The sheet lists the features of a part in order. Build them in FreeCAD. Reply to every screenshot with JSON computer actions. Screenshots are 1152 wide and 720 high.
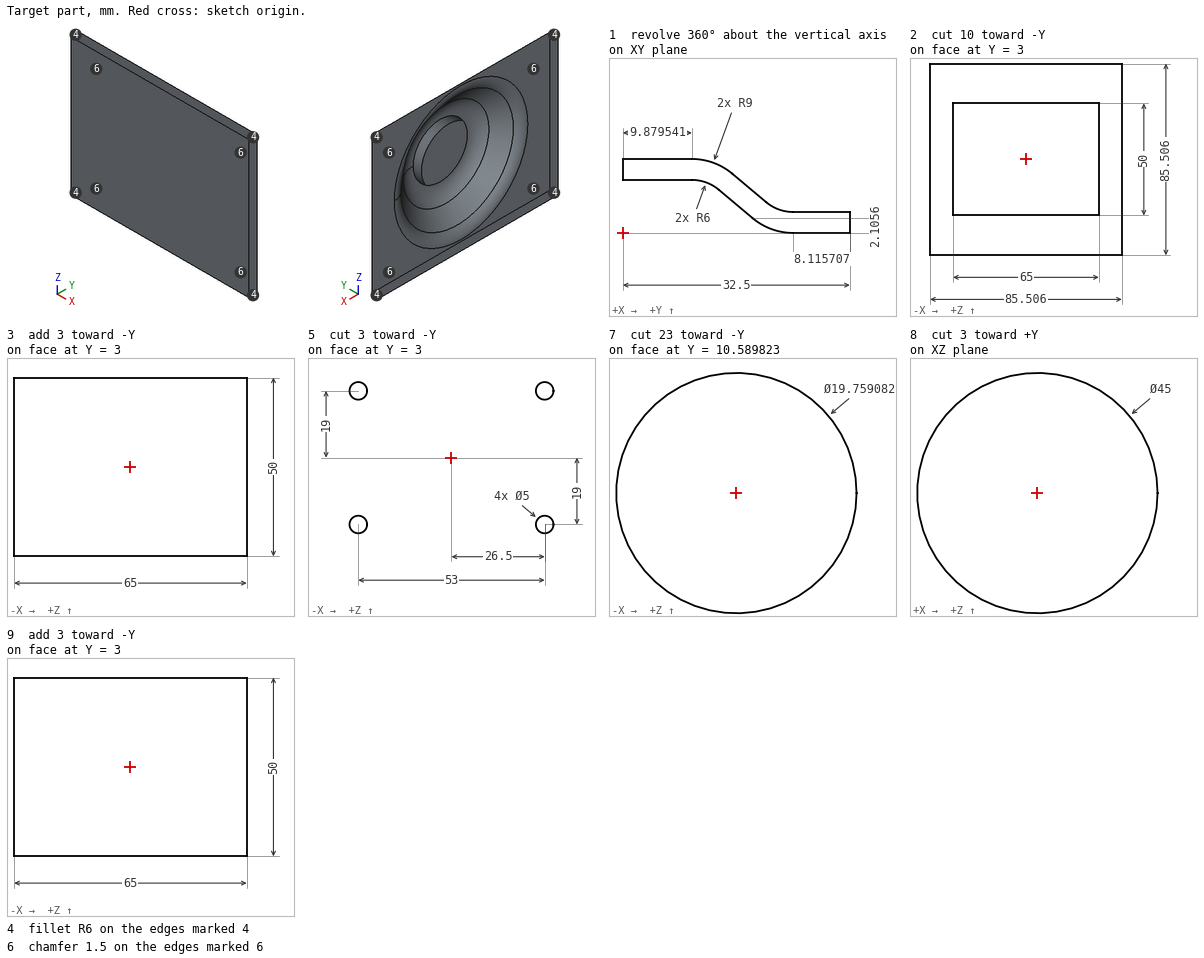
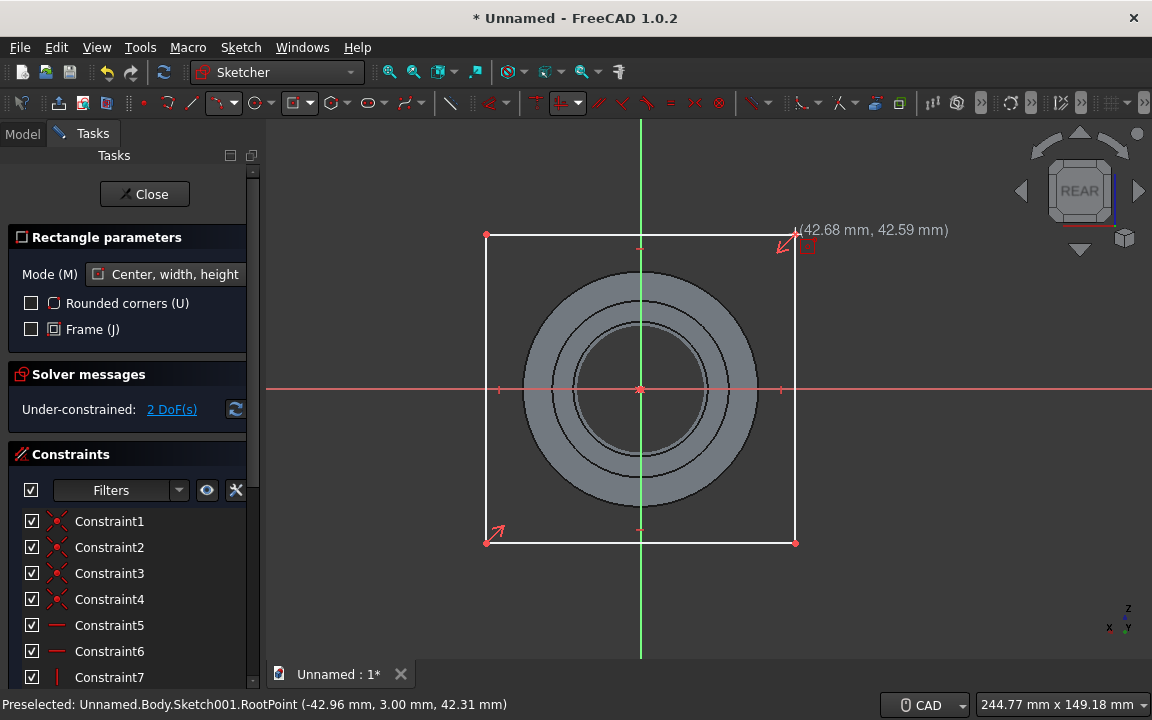
{"action": "left_click", "coordinate": [641, 389]}
{"action": "left_click", "coordinate": [758, 299]}
{"action": "key", "text": "Escape"}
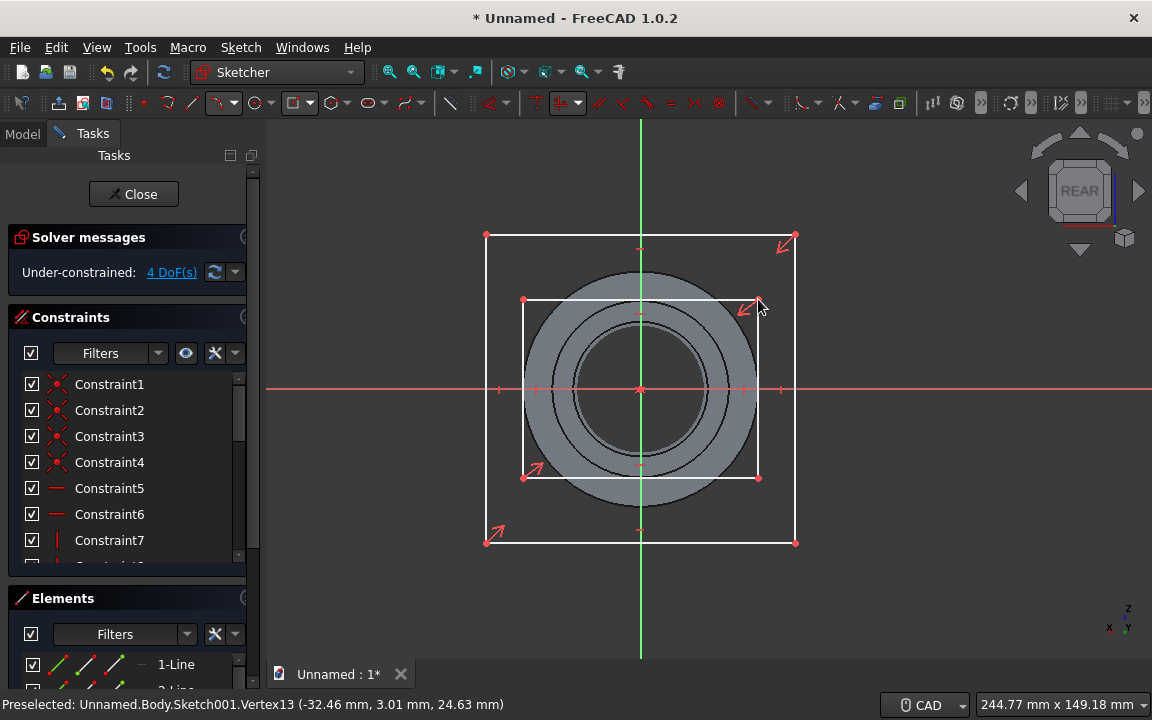
{"action": "left_click", "coordinate": [490, 104]}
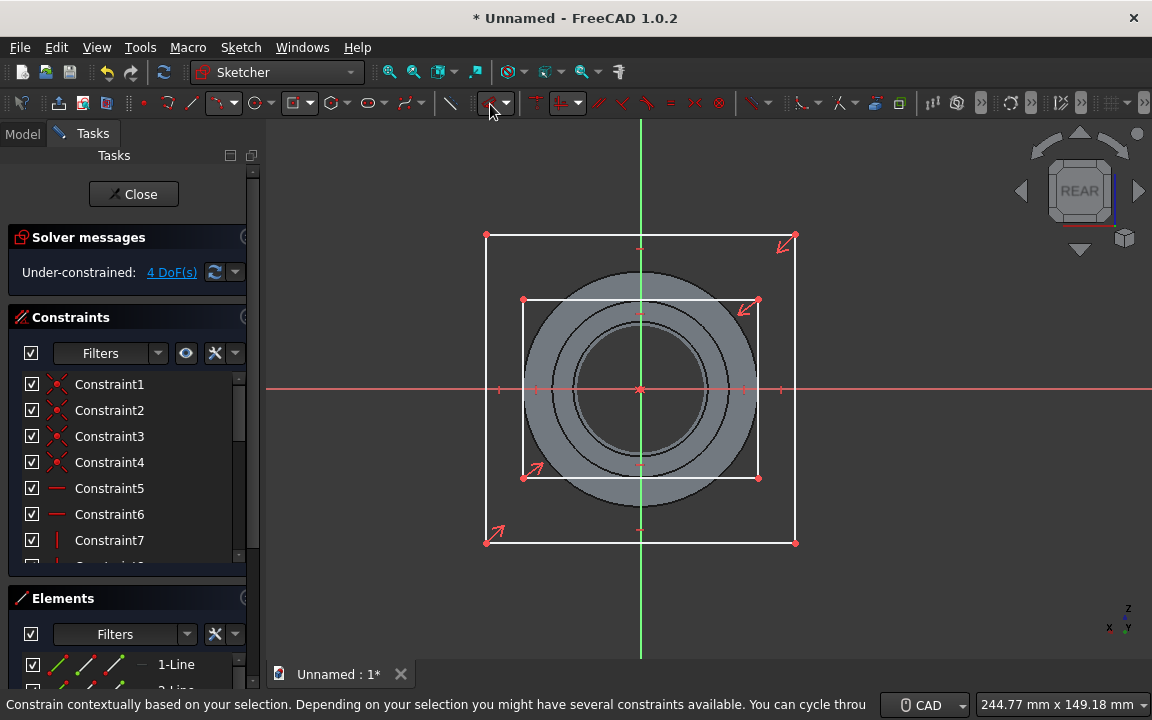
{"action": "left_click", "coordinate": [594, 478]}
{"action": "left_click", "coordinate": [586, 512]}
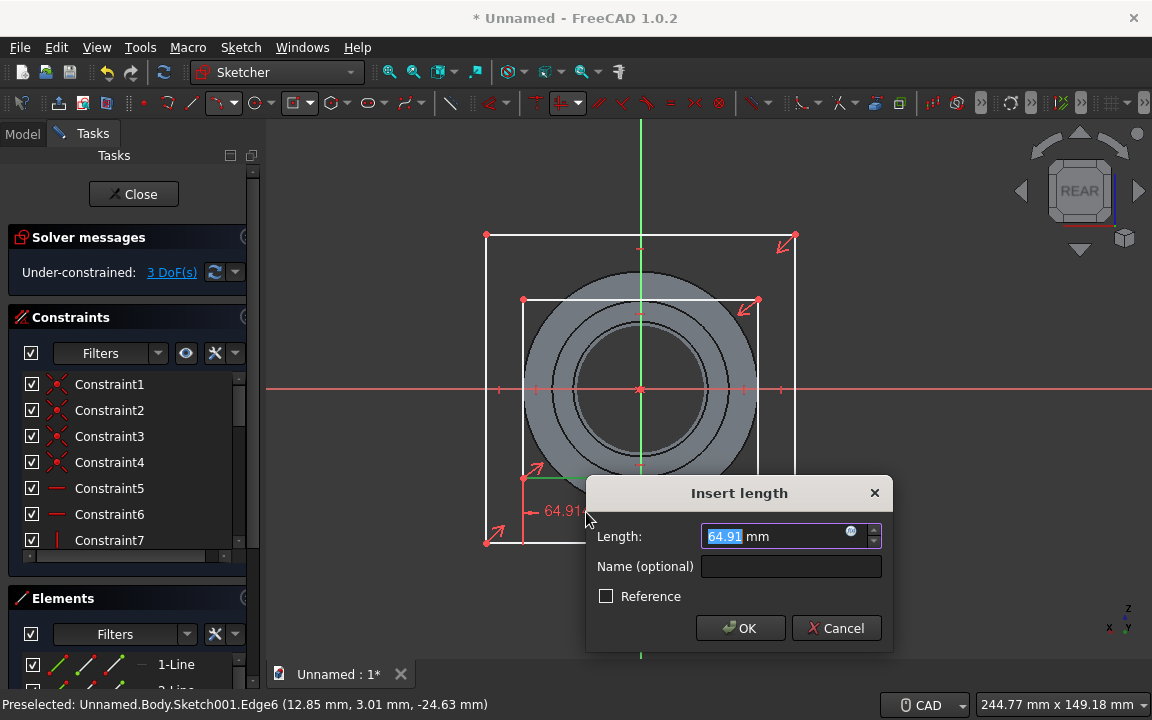
{"action": "type", "text": "65"}
{"action": "key", "text": "Return"}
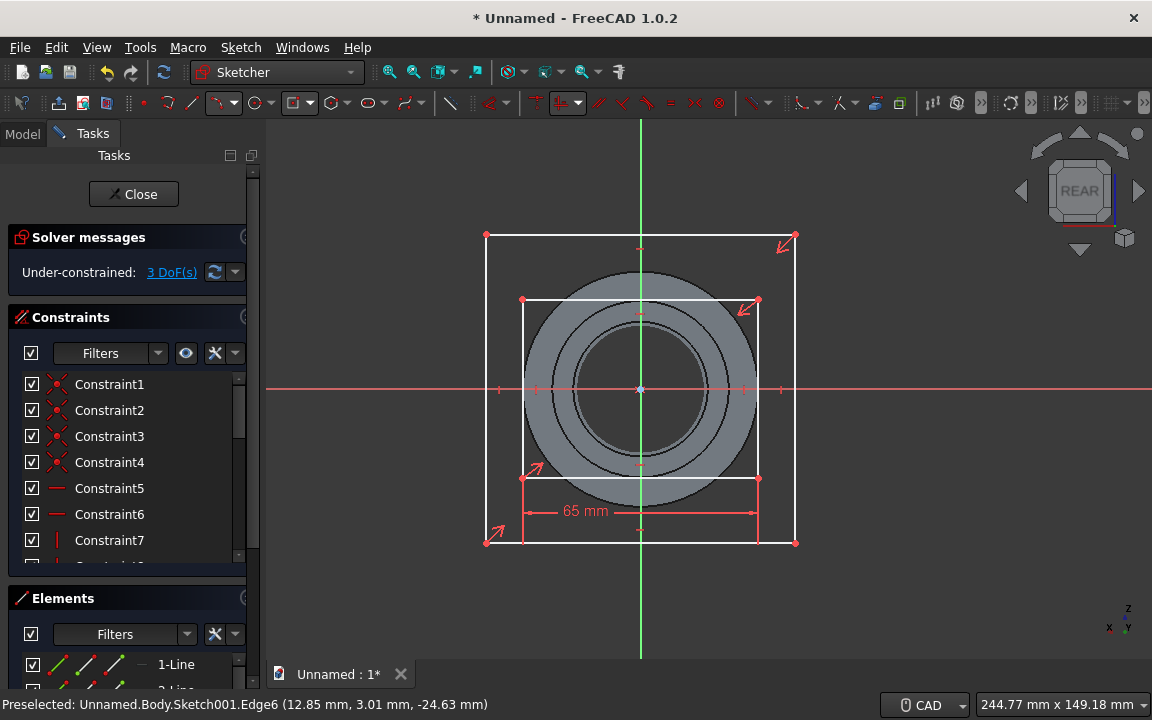
{"action": "left_click", "coordinate": [758, 425]}
{"action": "left_click", "coordinate": [724, 348]}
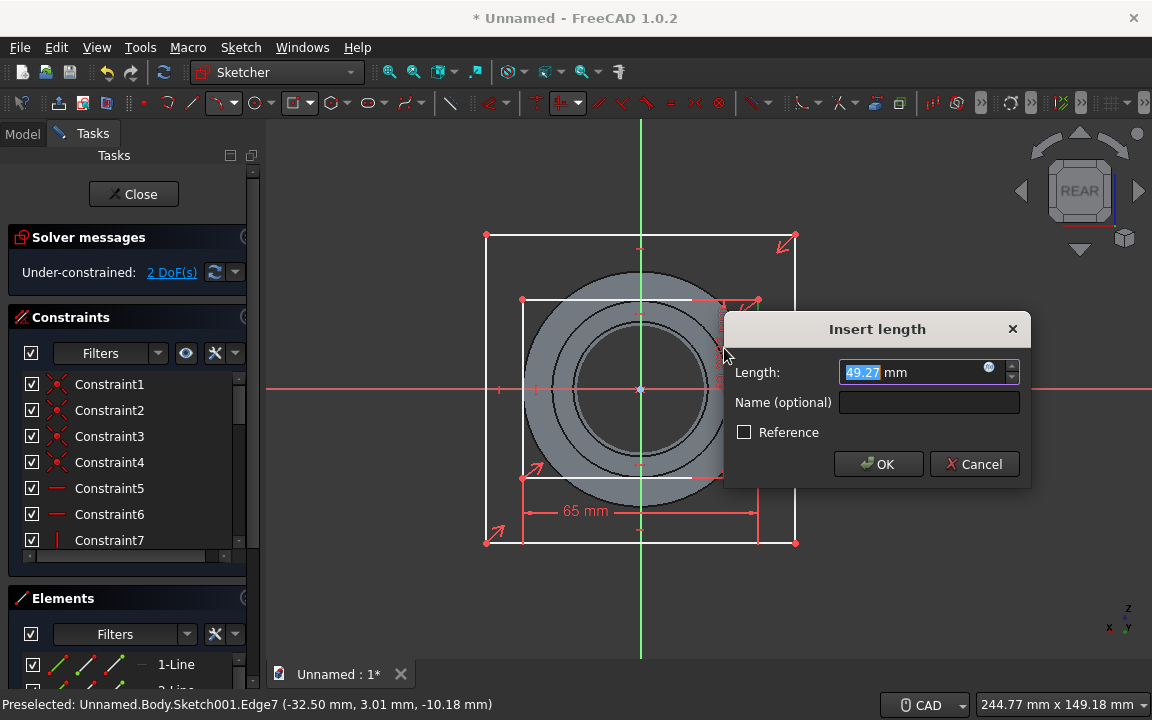
{"action": "type", "text": "50"}
{"action": "key", "text": "Return"}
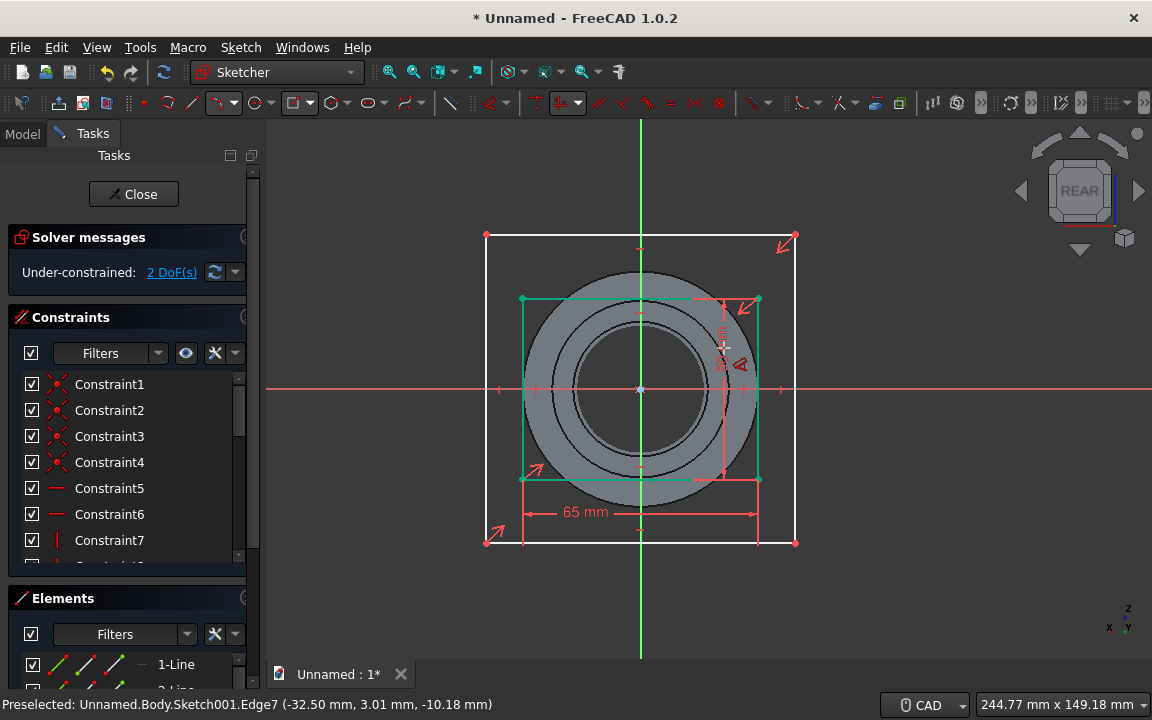
{"action": "left_click", "coordinate": [579, 543]}
{"action": "left_click", "coordinate": [569, 577]}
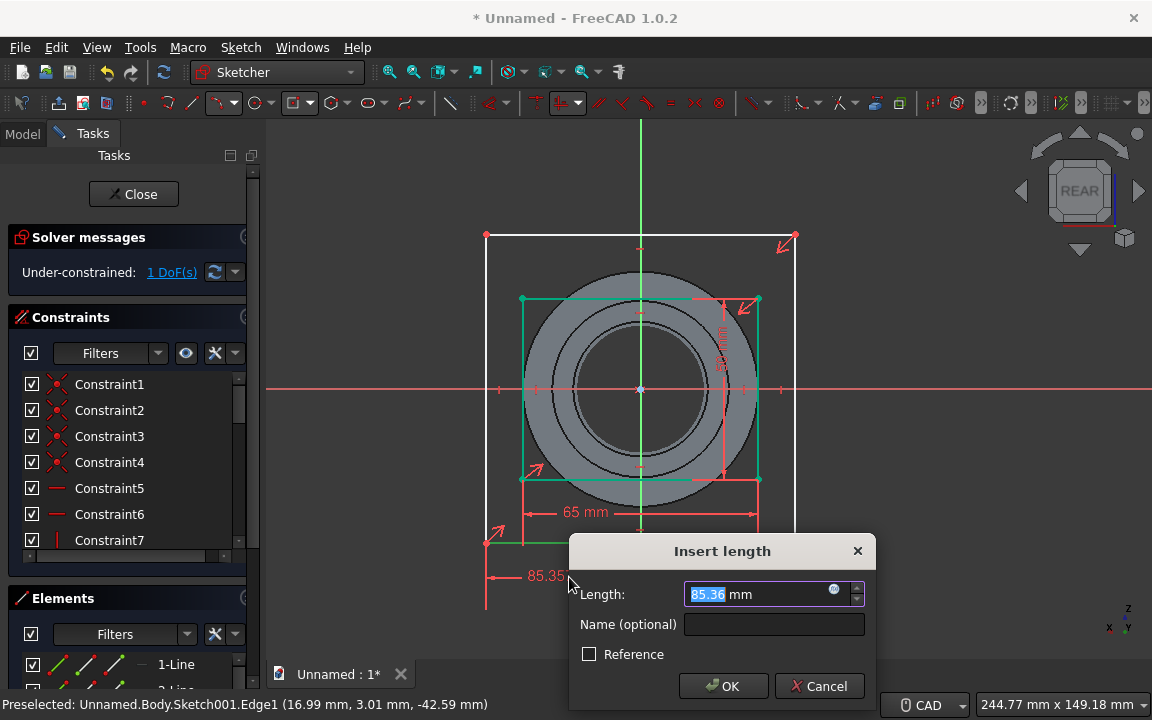
{"action": "type", "text": "85.506"}
{"action": "key", "text": "Return"}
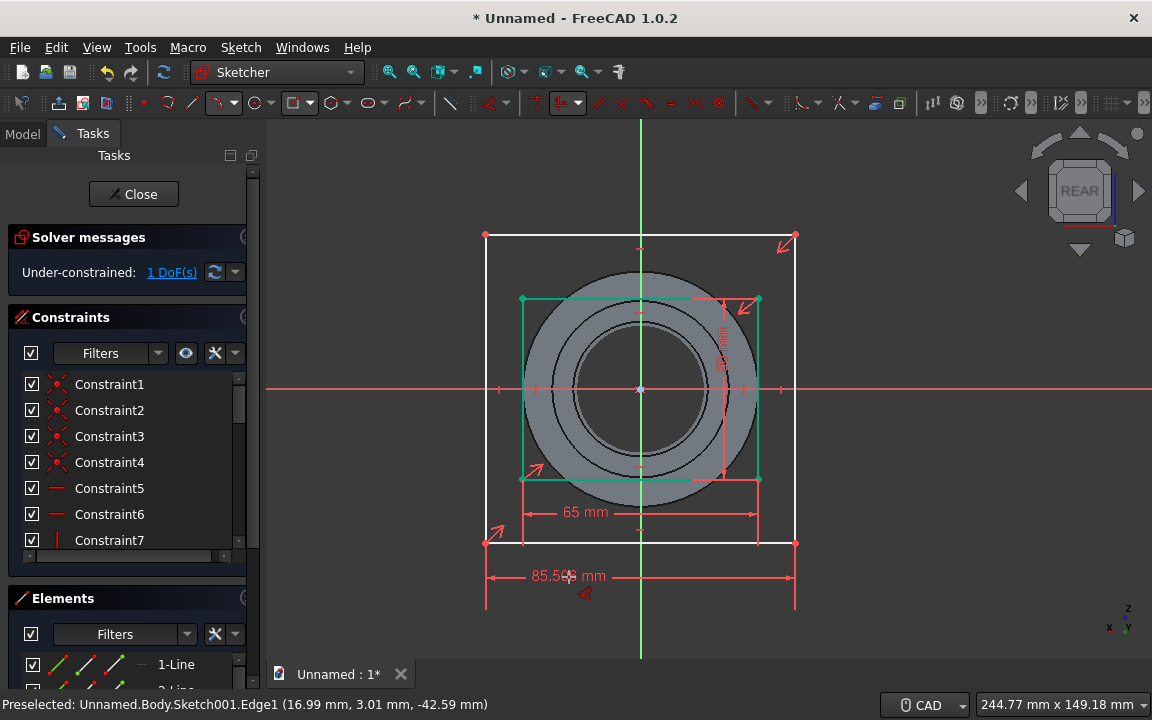
{"action": "left_click", "coordinate": [795, 451]}
{"action": "left_click", "coordinate": [829, 318]}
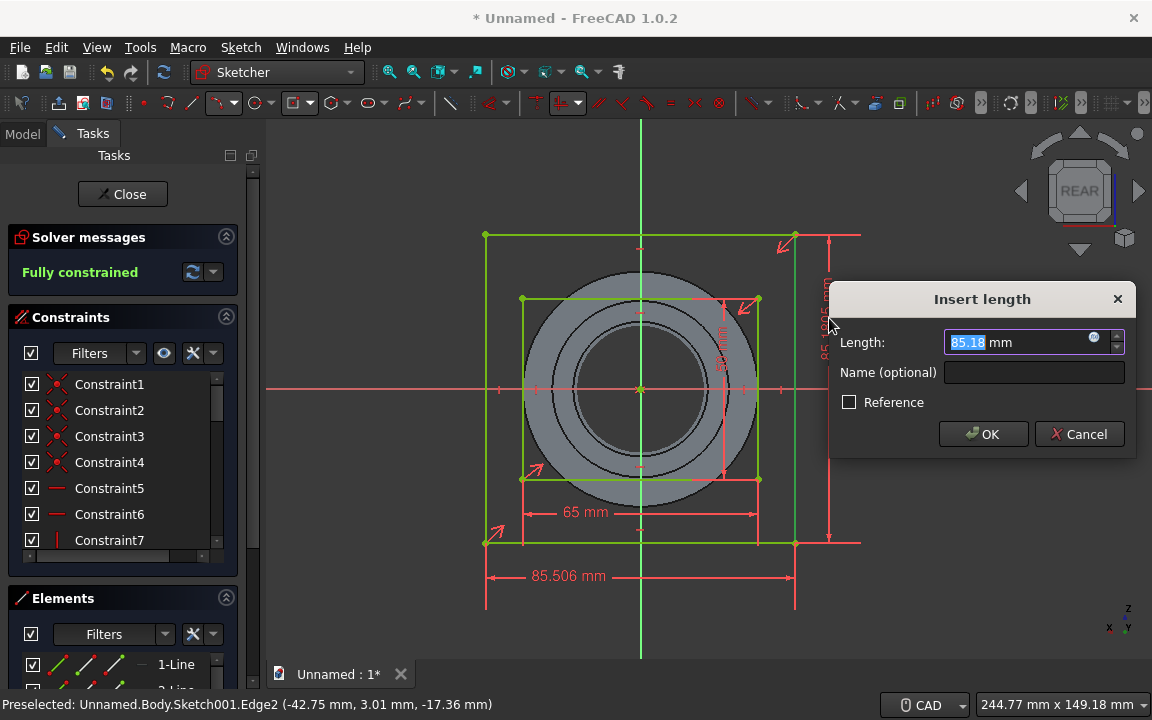
{"action": "type", "text": "85.506"}
{"action": "key", "text": "Return"}
{"action": "key", "text": "Escape"}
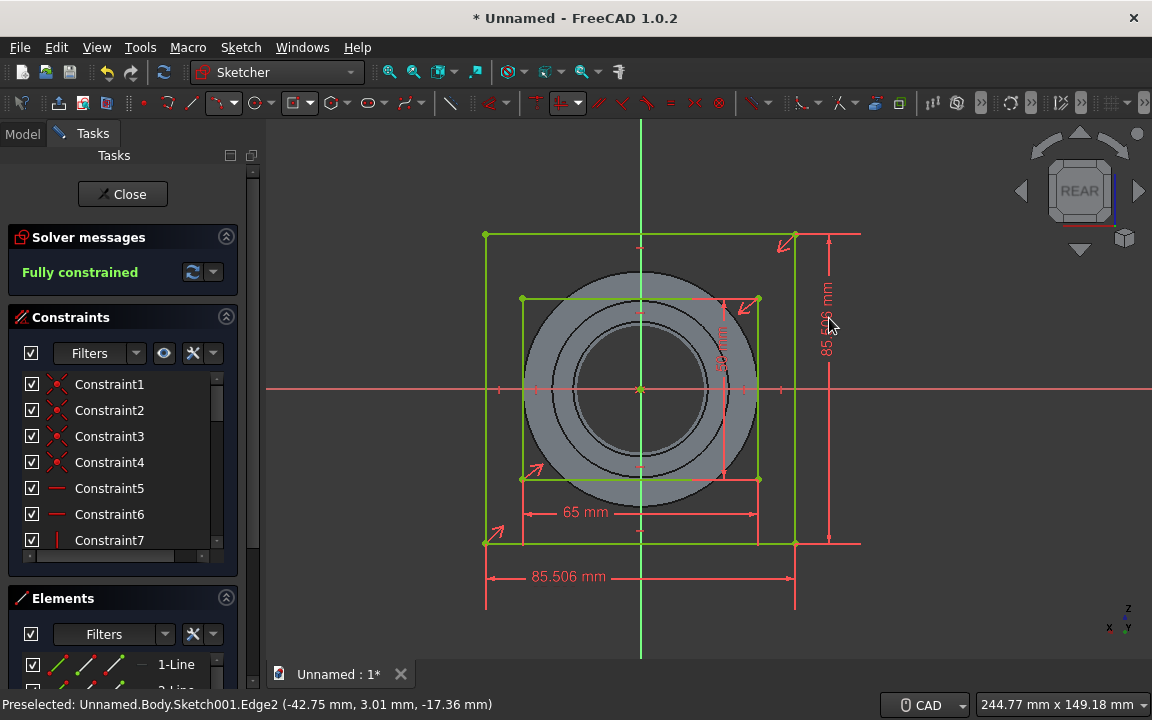
{"action": "left_click", "coordinate": [123, 194]}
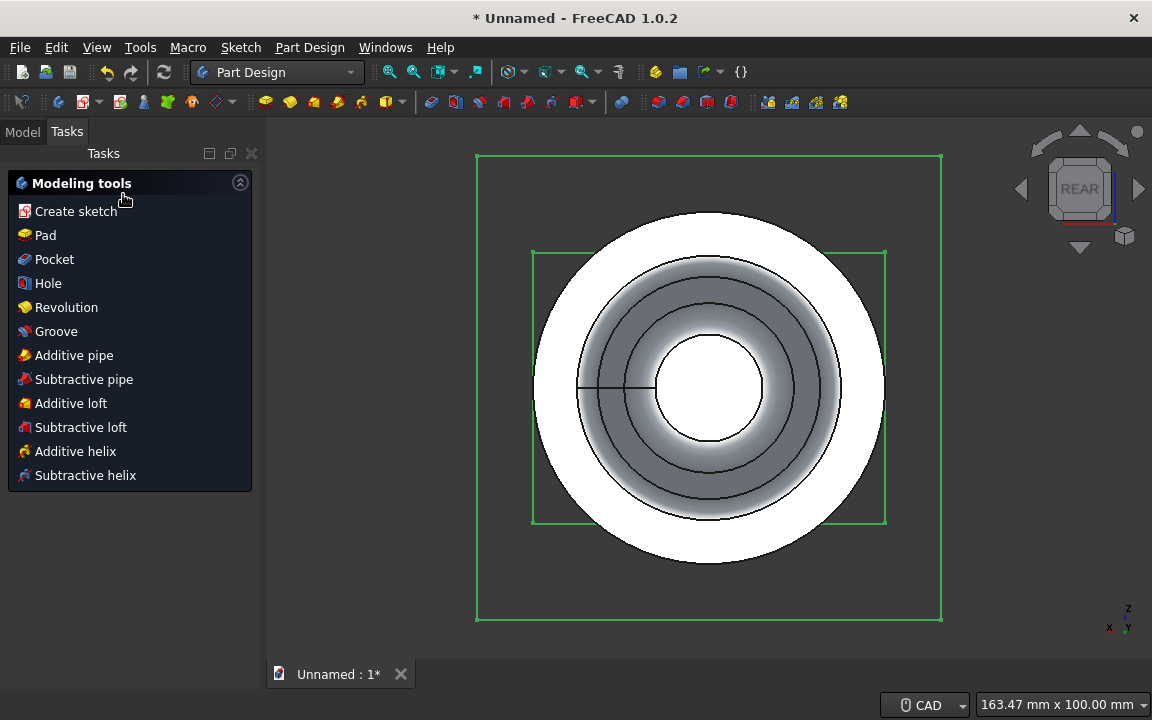
{"action": "left_click", "coordinate": [432, 102]}